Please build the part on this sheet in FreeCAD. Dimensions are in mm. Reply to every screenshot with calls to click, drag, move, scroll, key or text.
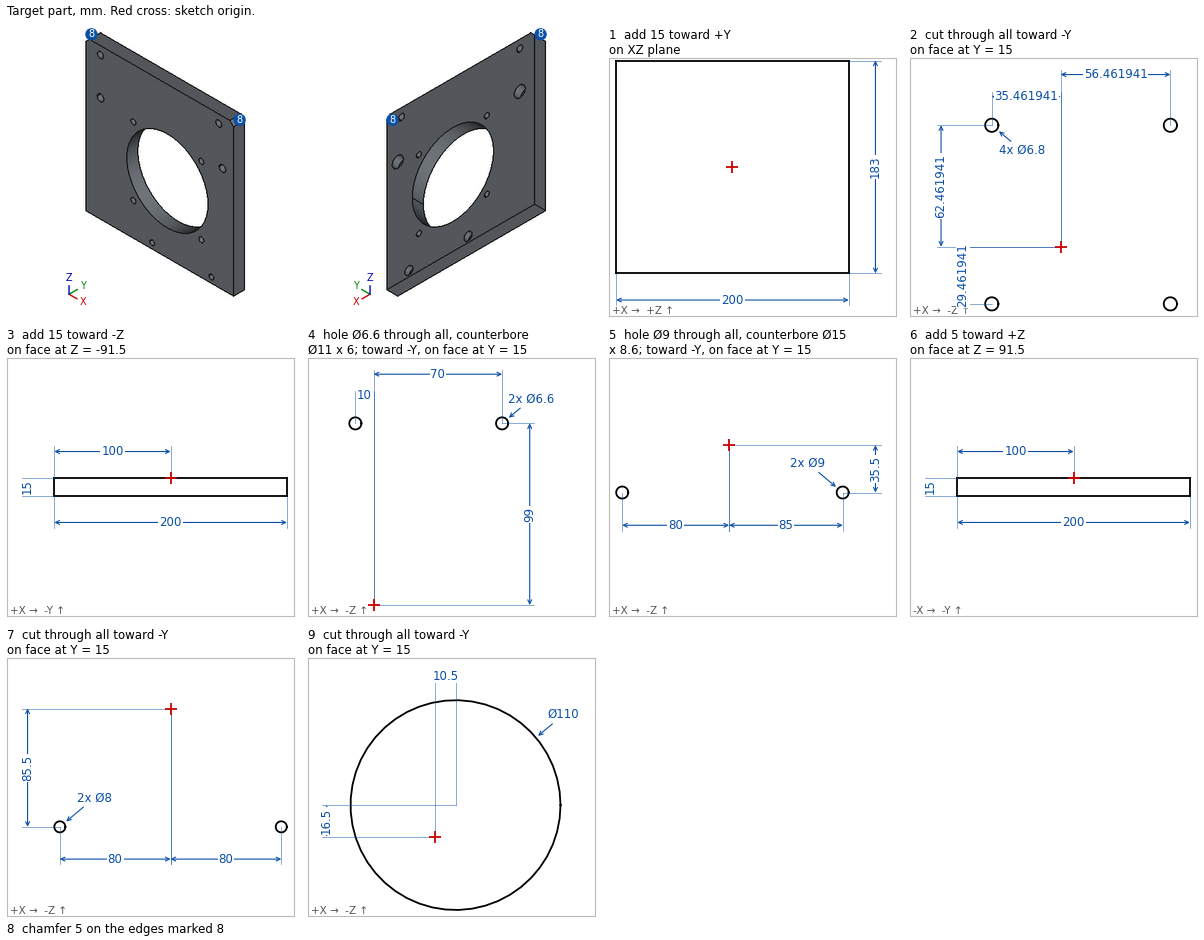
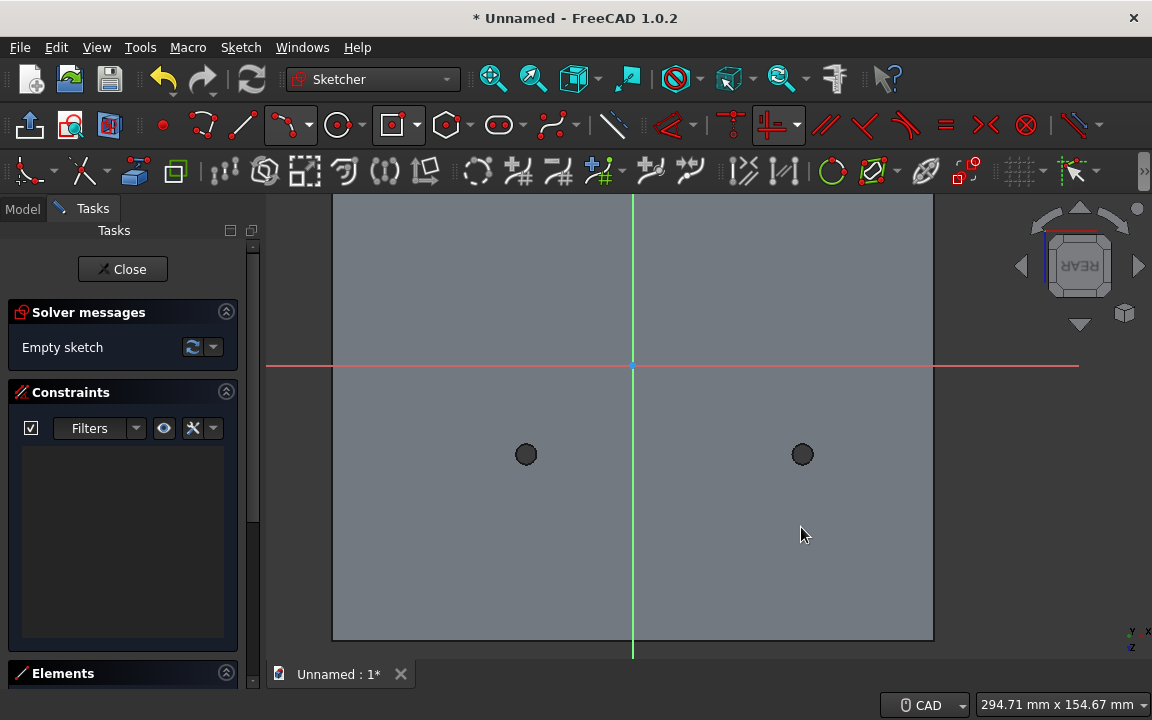
click(338, 126)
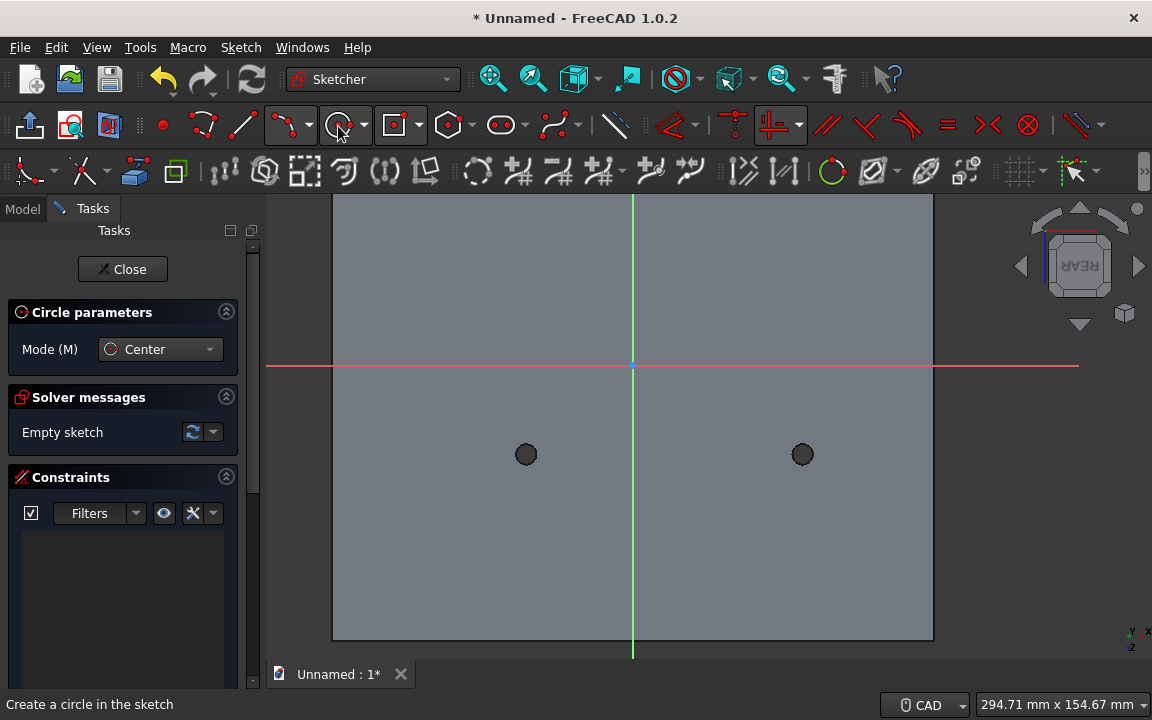
scroll(888, 473, up, 3)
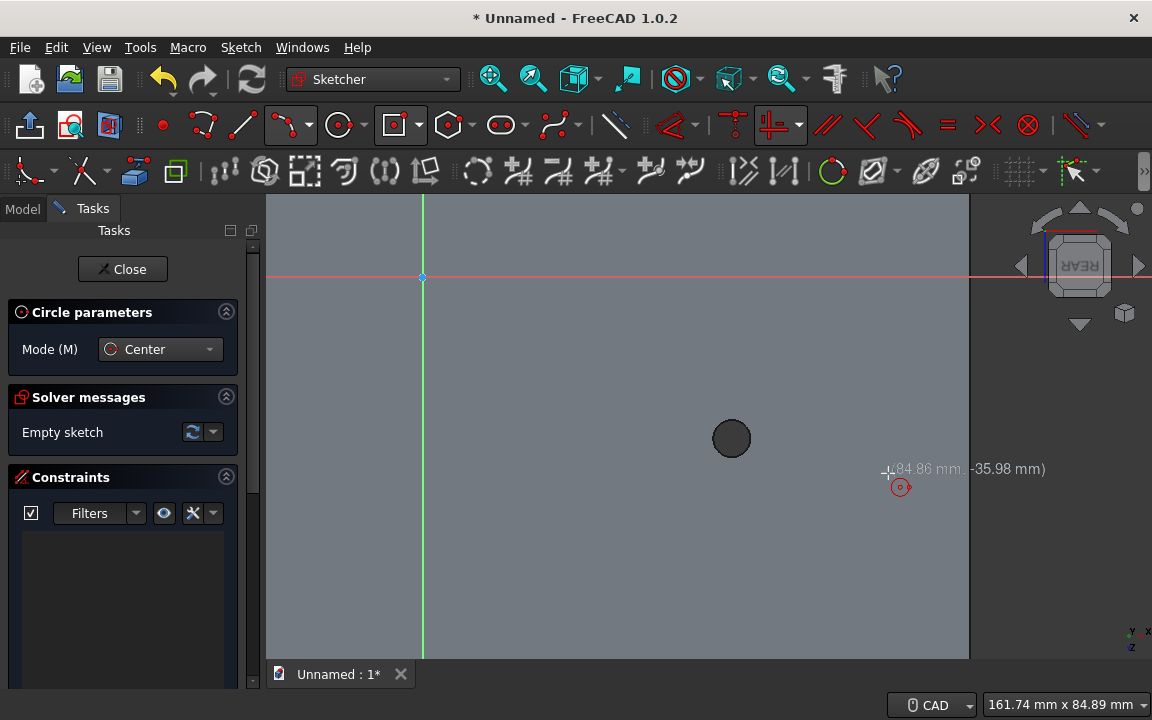
click(888, 472)
click(906, 454)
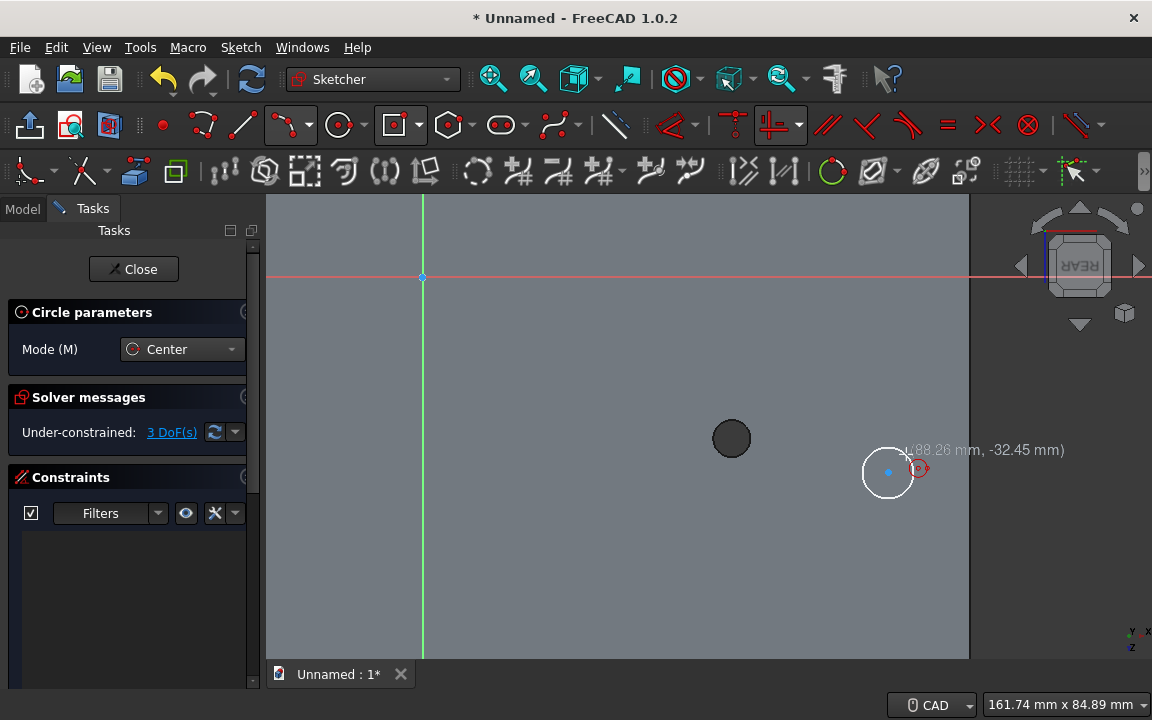
scroll(889, 475, down, 3)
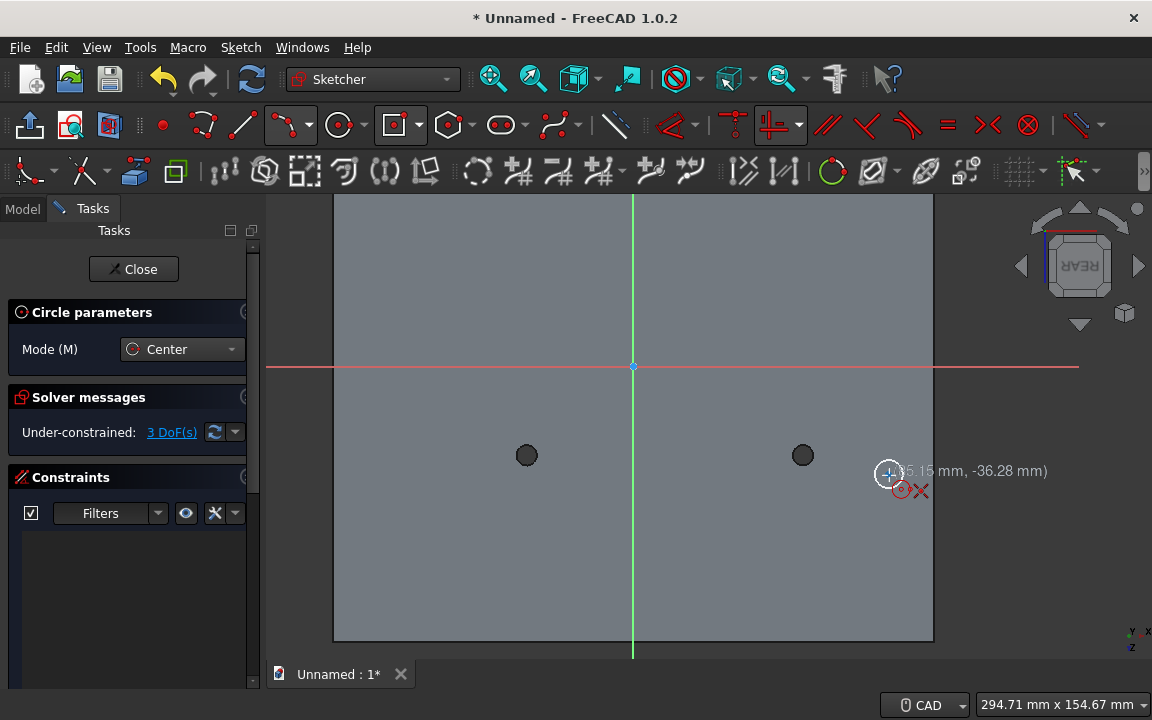
scroll(393, 473, up, 3)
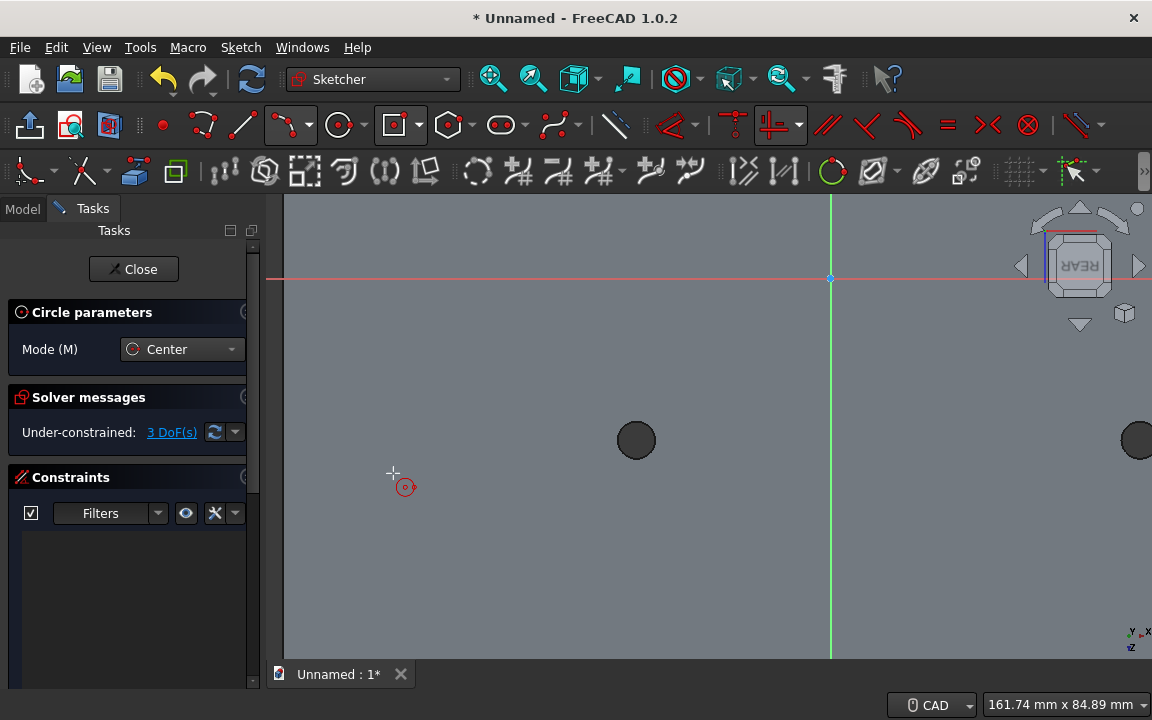
click(393, 473)
click(410, 456)
key(Escape)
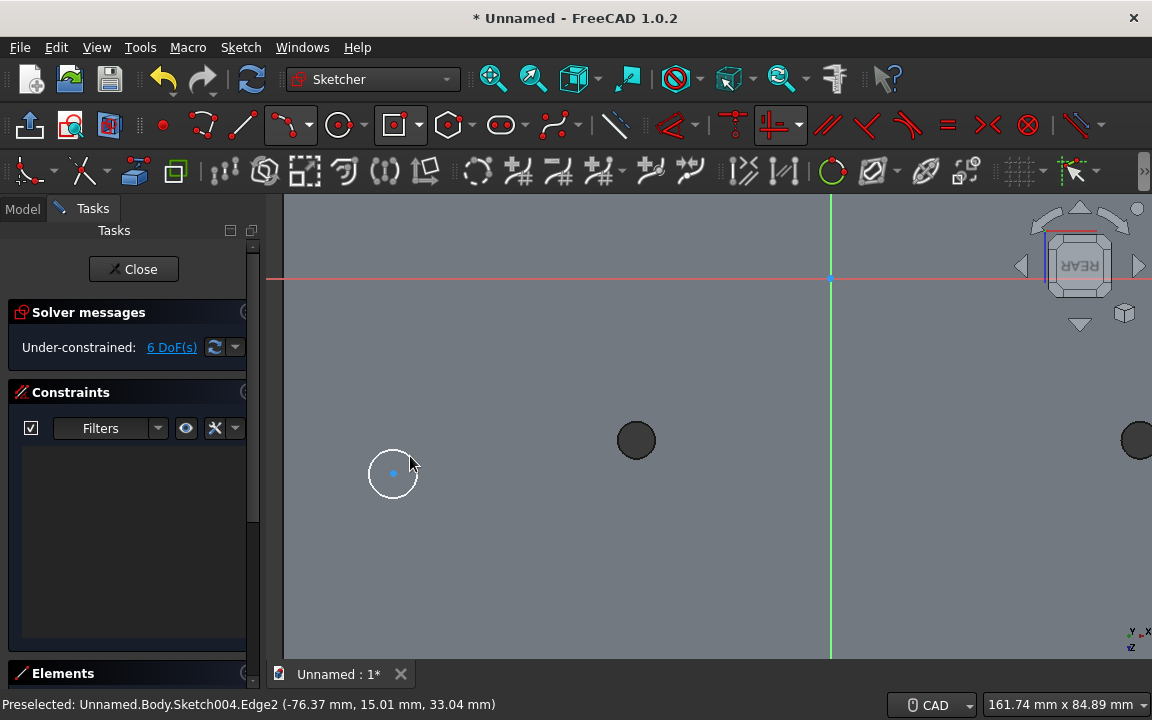
scroll(392, 473, down, 3)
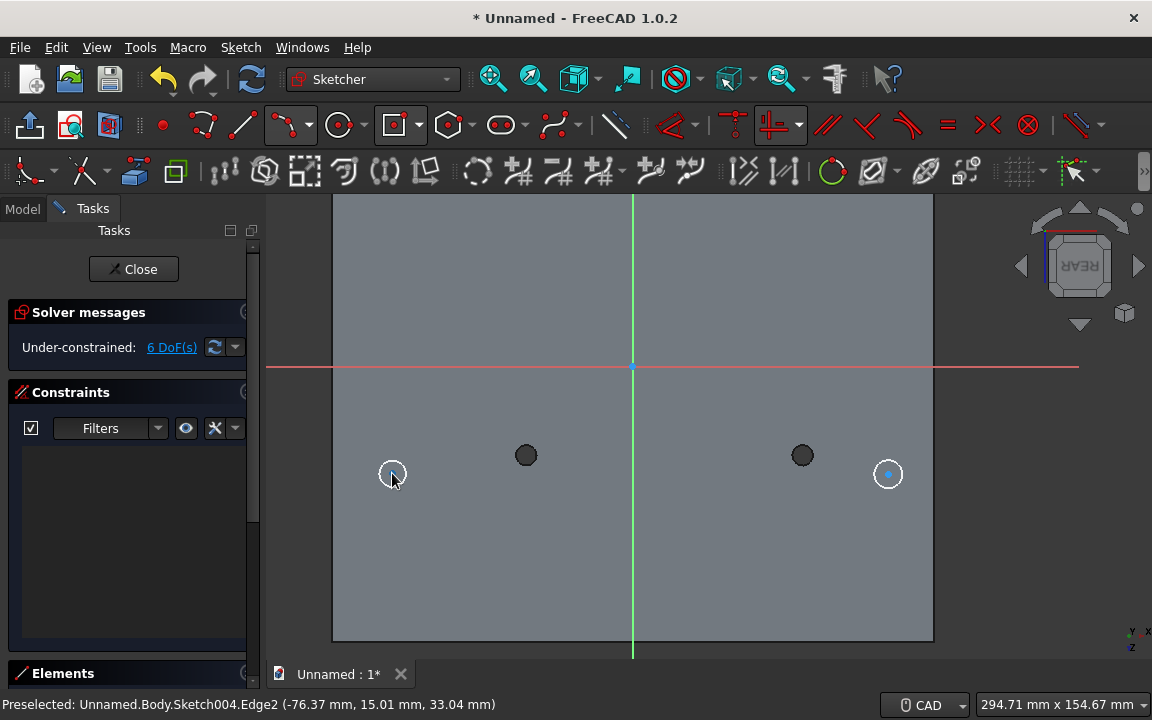
click(898, 464)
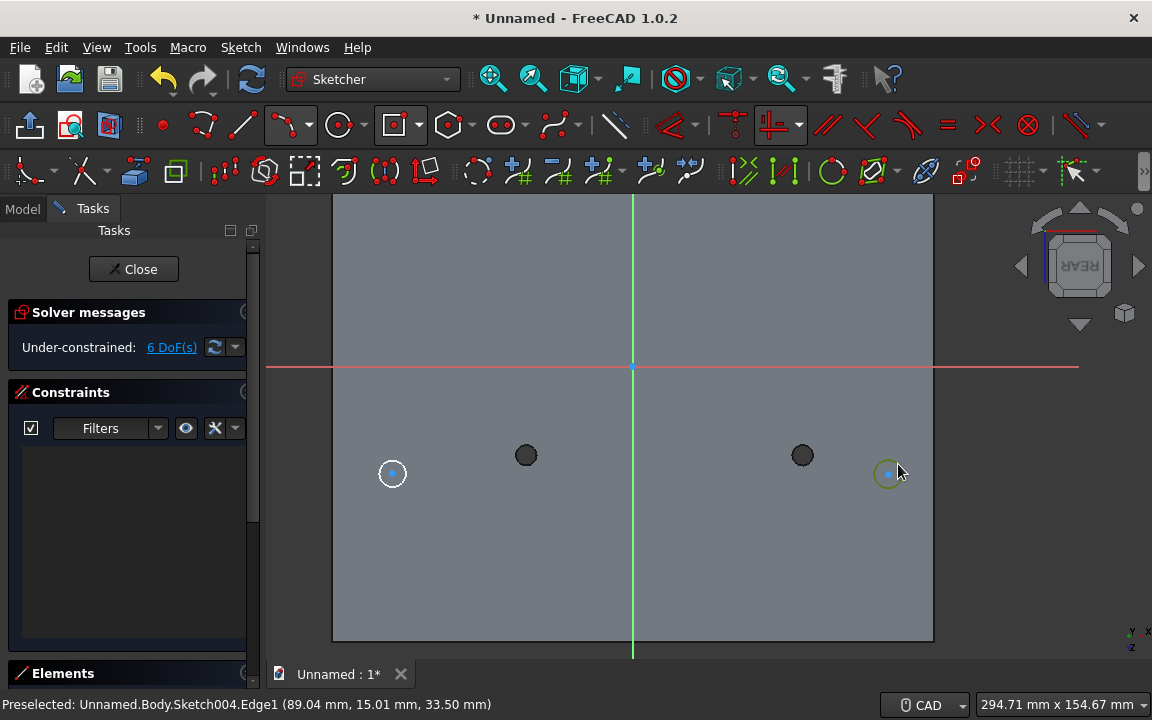
click(402, 464)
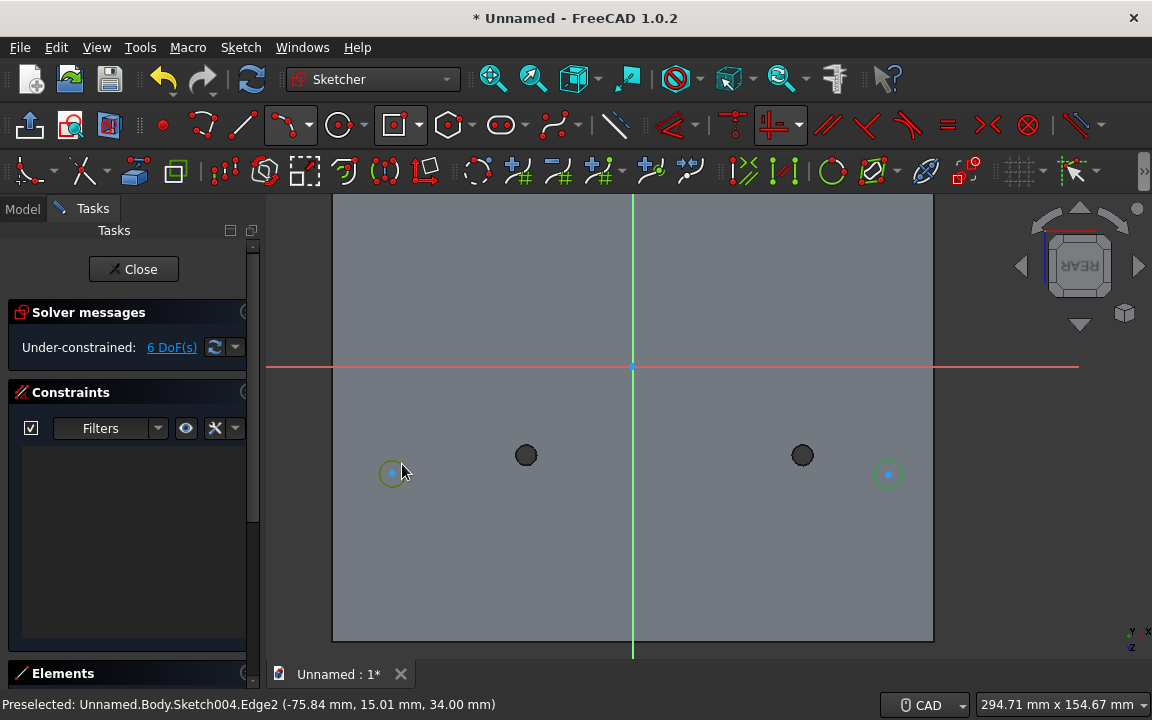
click(948, 126)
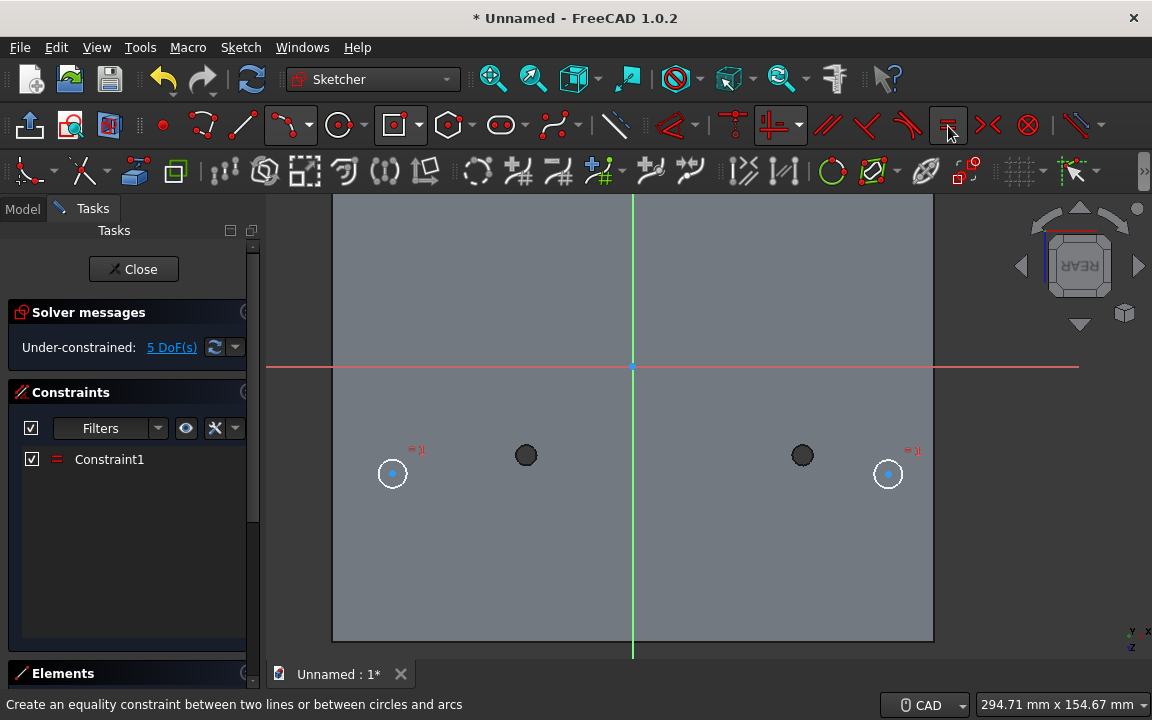
click(888, 474)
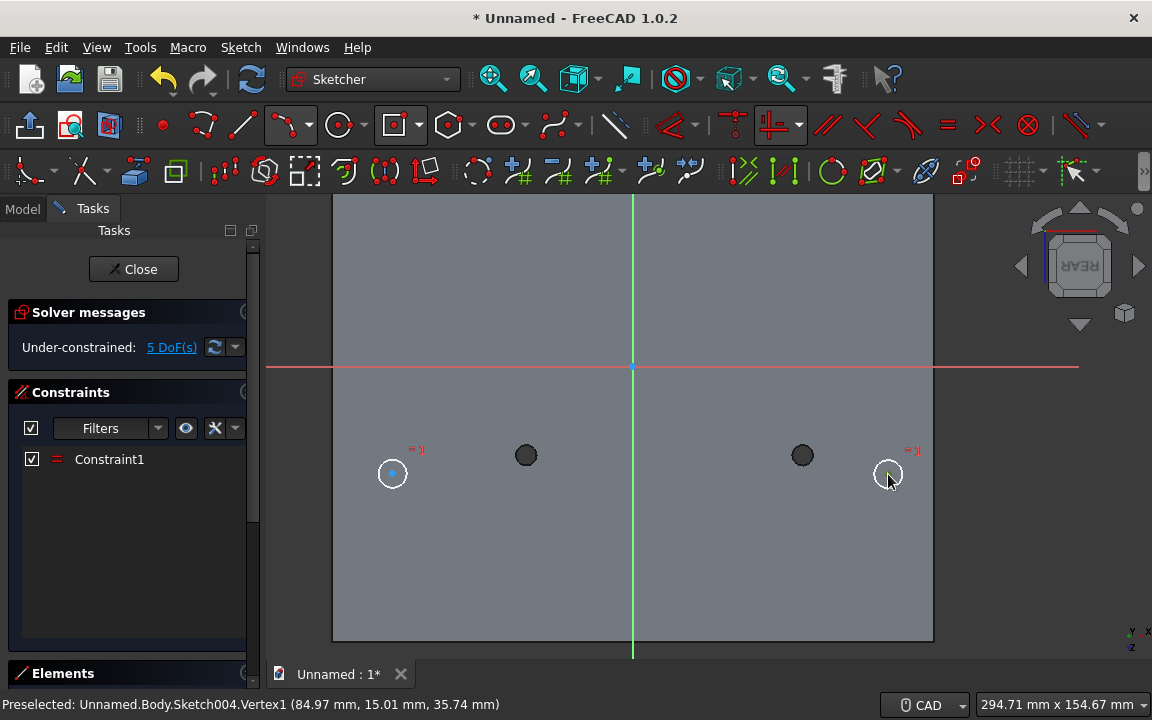
click(393, 474)